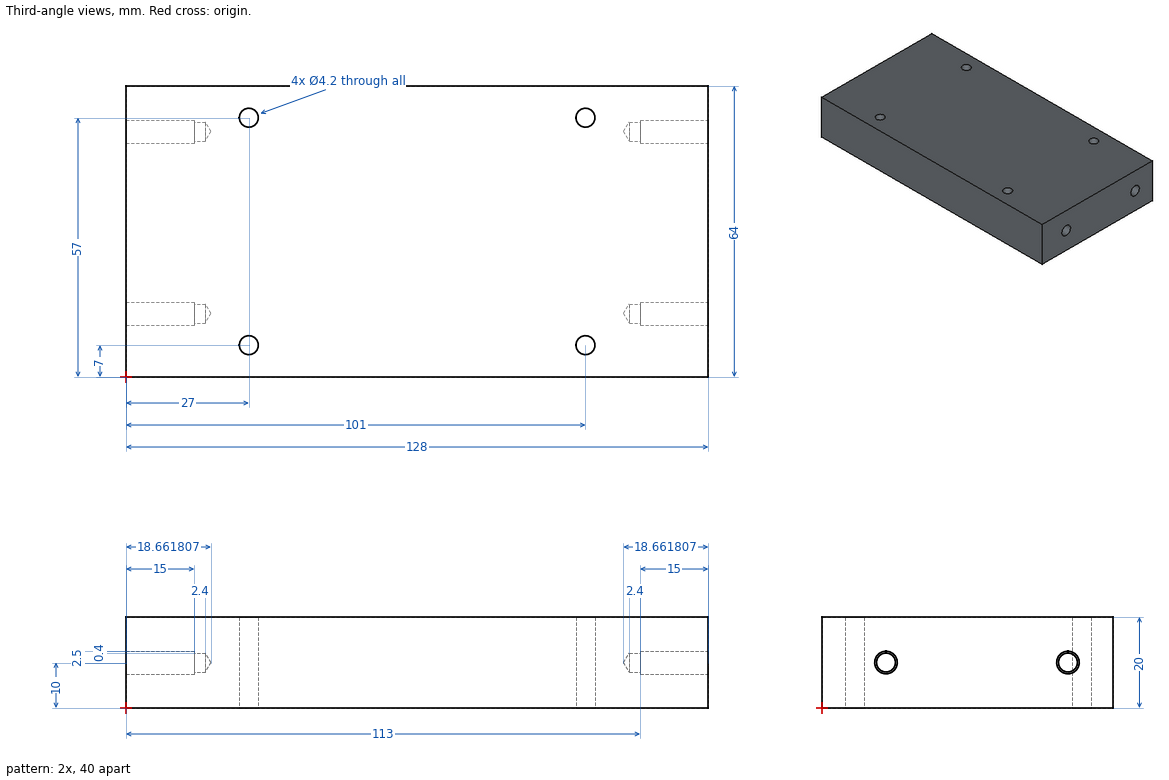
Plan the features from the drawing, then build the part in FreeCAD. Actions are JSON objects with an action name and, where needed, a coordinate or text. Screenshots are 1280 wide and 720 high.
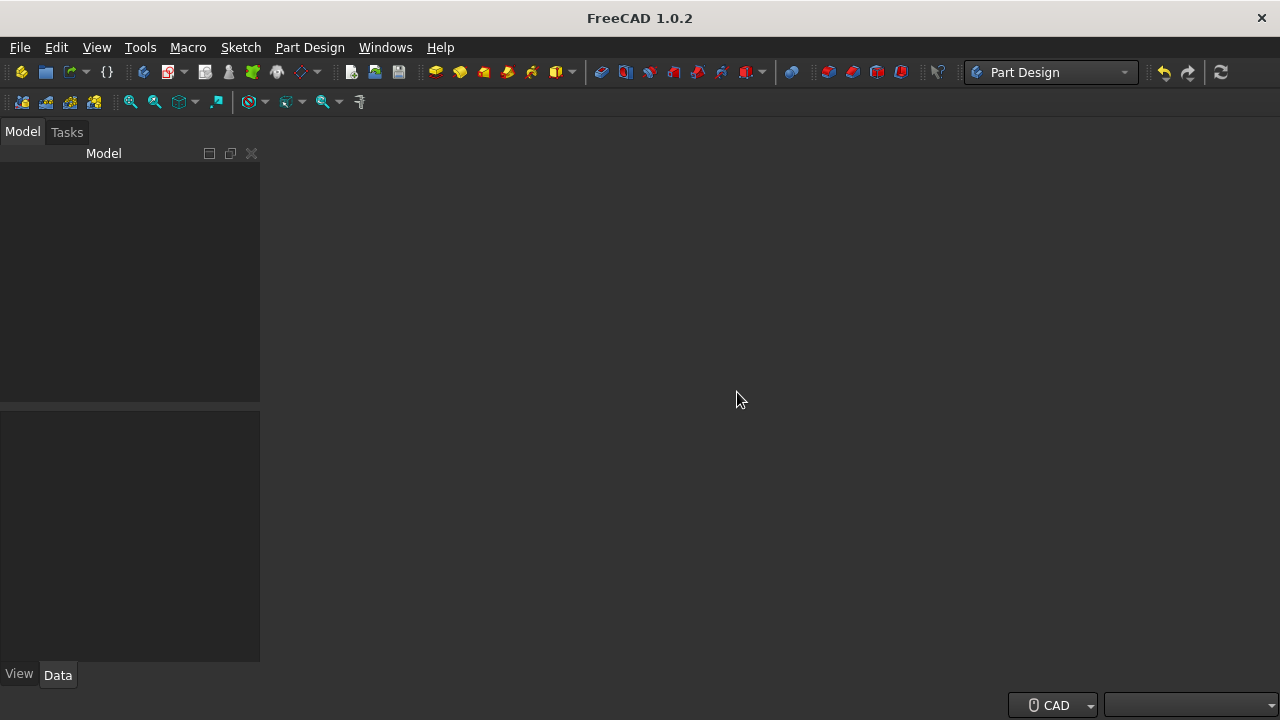
{"action": "left_click", "coordinate": [352, 72]}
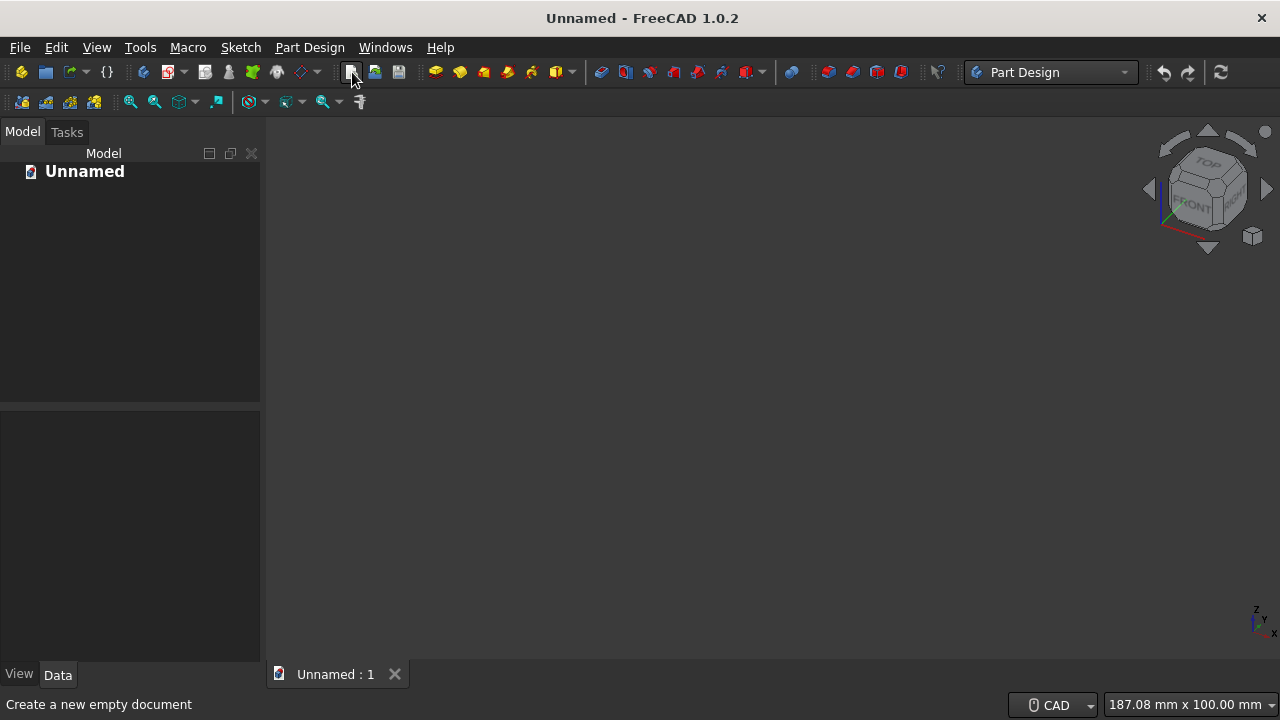
{"action": "left_click", "coordinate": [168, 72]}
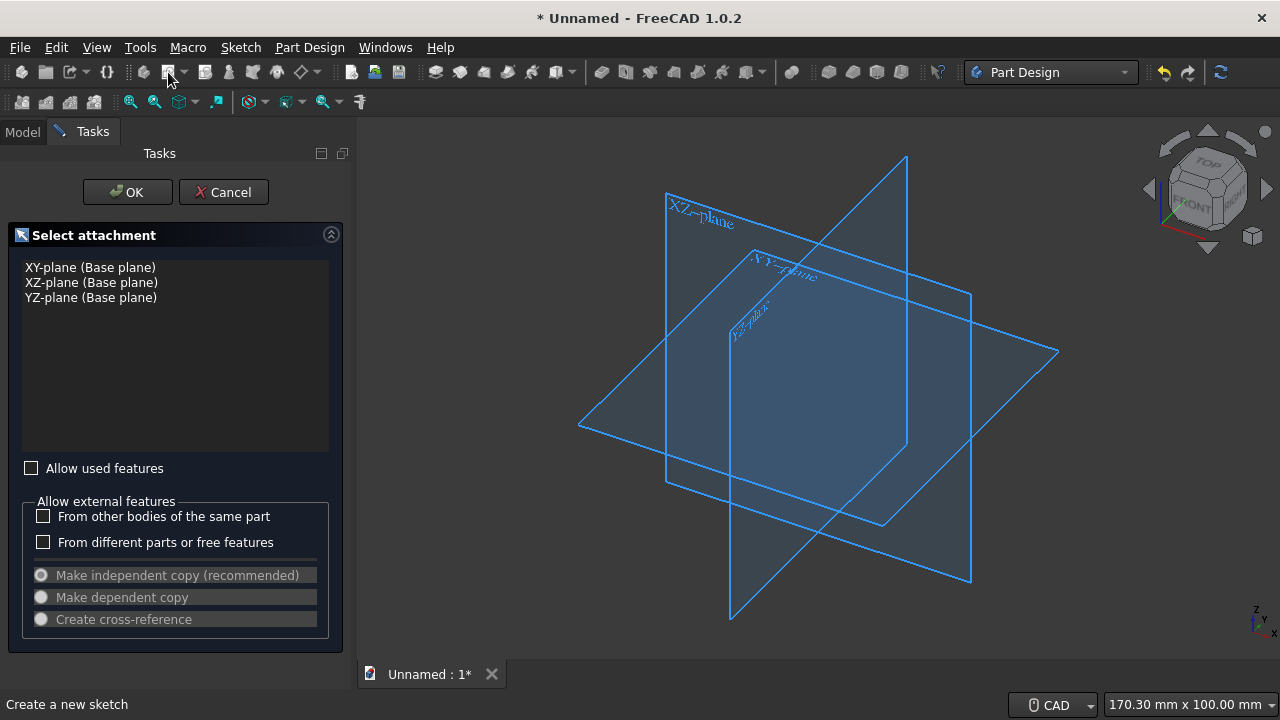
{"action": "left_click", "coordinate": [82, 268]}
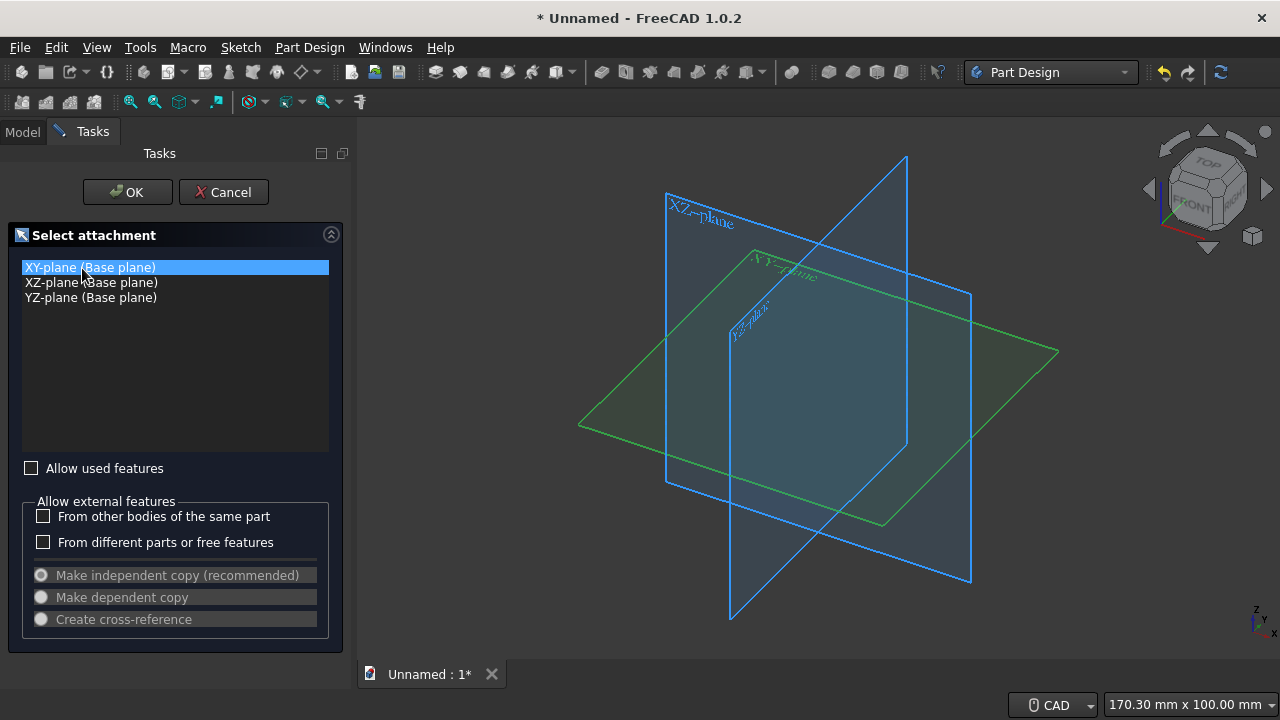
{"action": "left_click", "coordinate": [128, 192]}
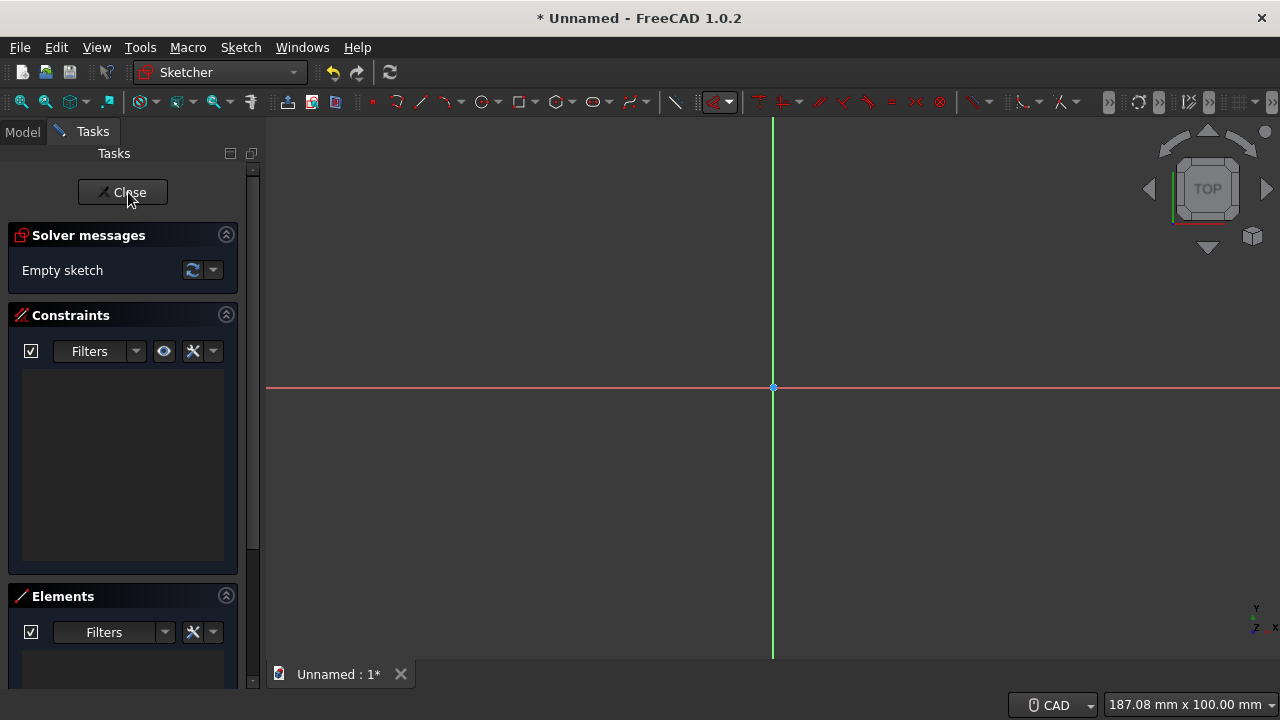
{"action": "scroll", "coordinate": [294, 631], "scroll_direction": "down", "scroll_amount": 2}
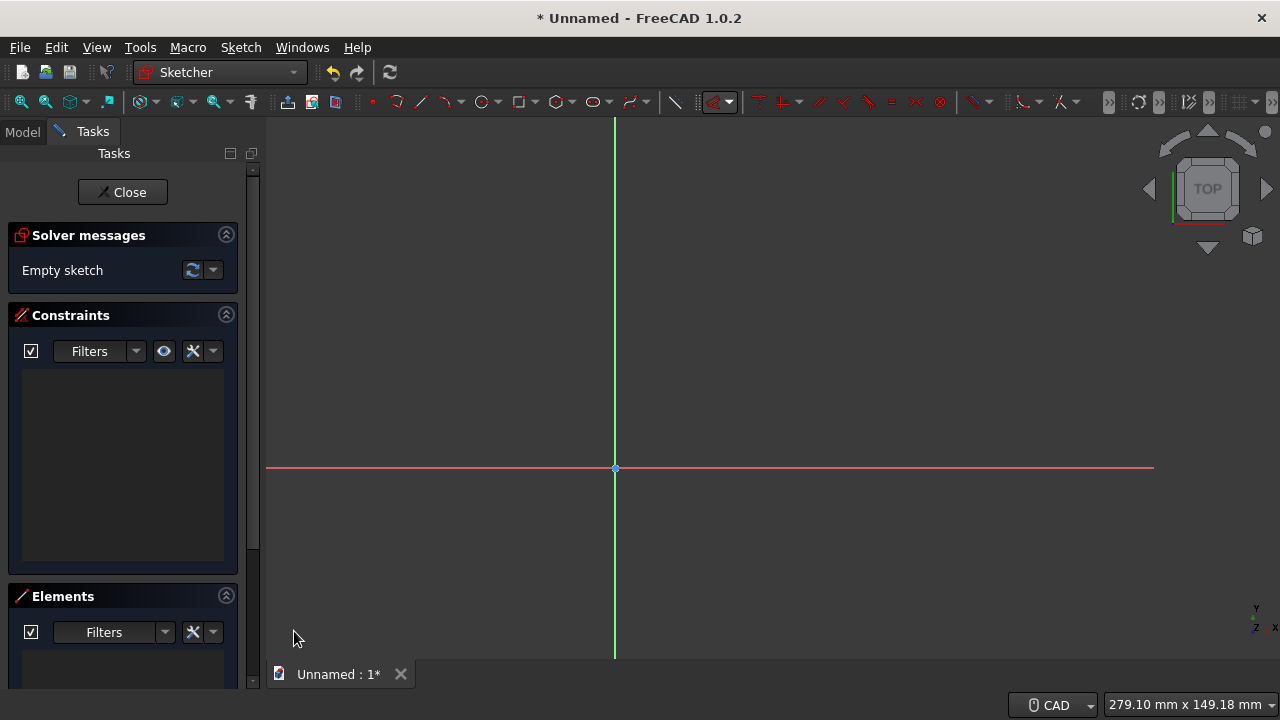
{"action": "left_click", "coordinate": [520, 102]}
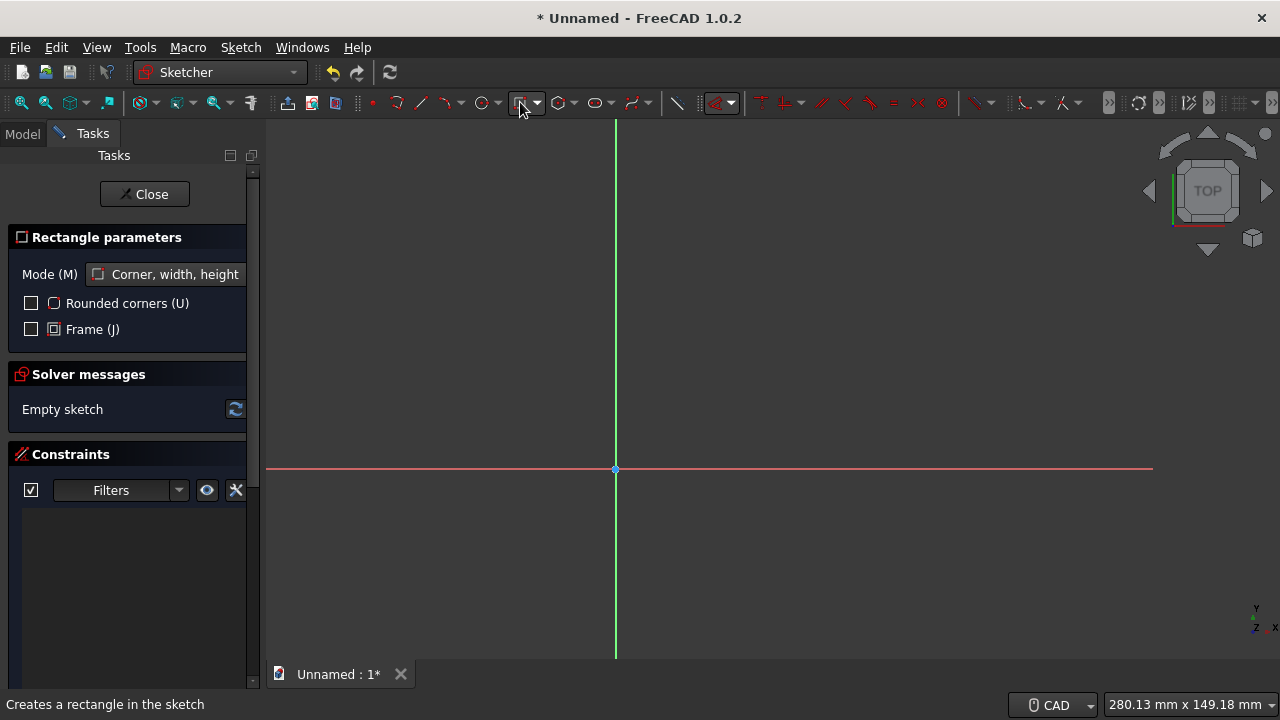
{"action": "left_click", "coordinate": [616, 469]}
{"action": "left_click", "coordinate": [1079, 237]}
{"action": "key", "text": "Escape"}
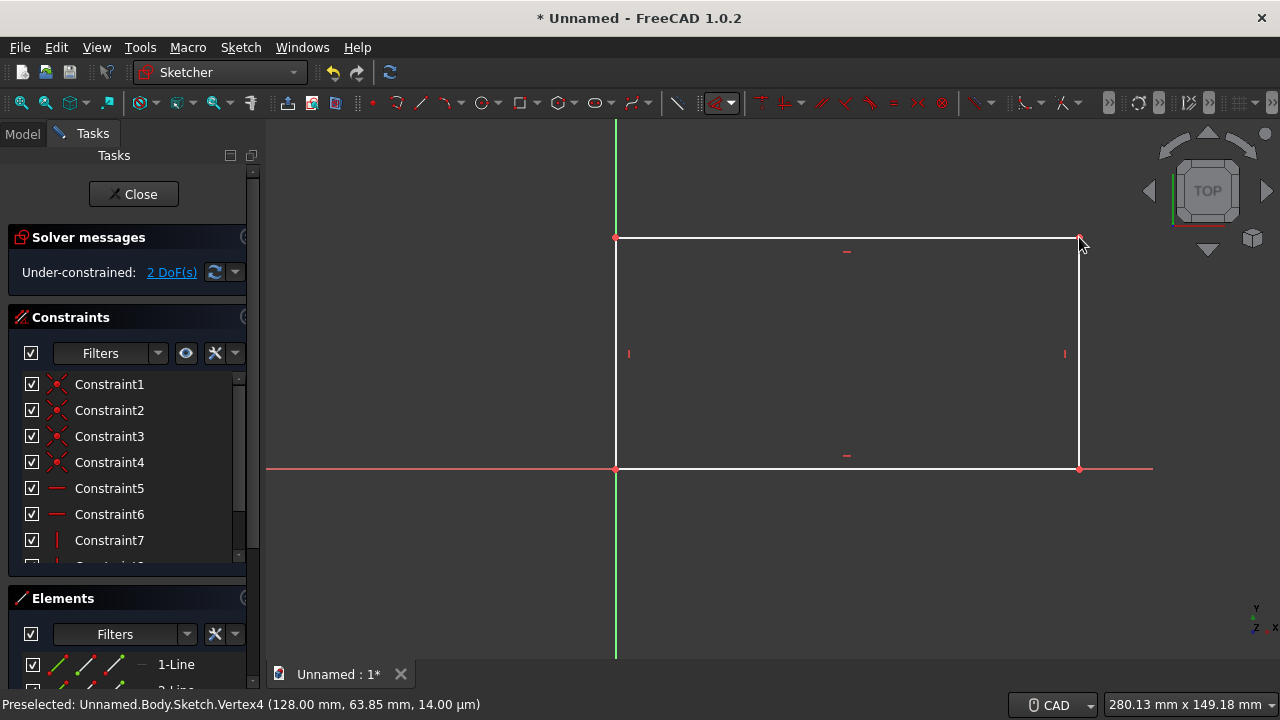
{"action": "left_click", "coordinate": [1079, 400]}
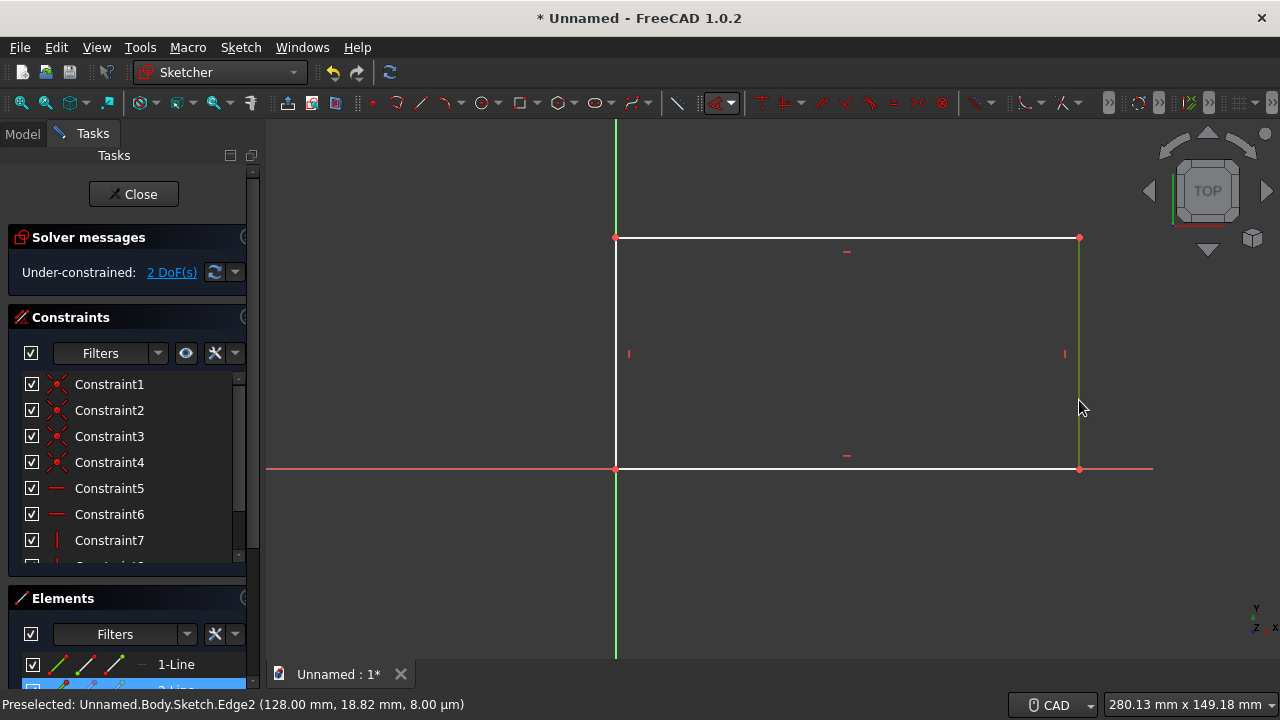
{"action": "key", "text": "i"}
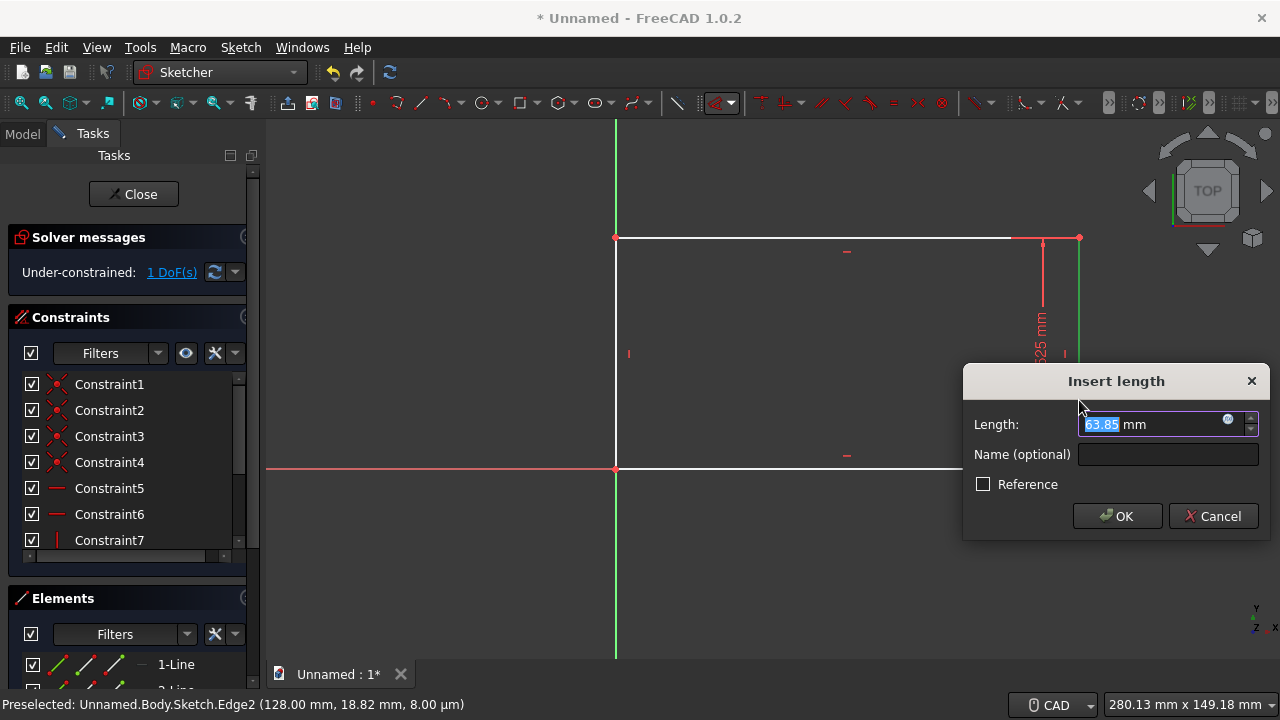
{"action": "type", "text": "64"}
{"action": "key", "text": "Return"}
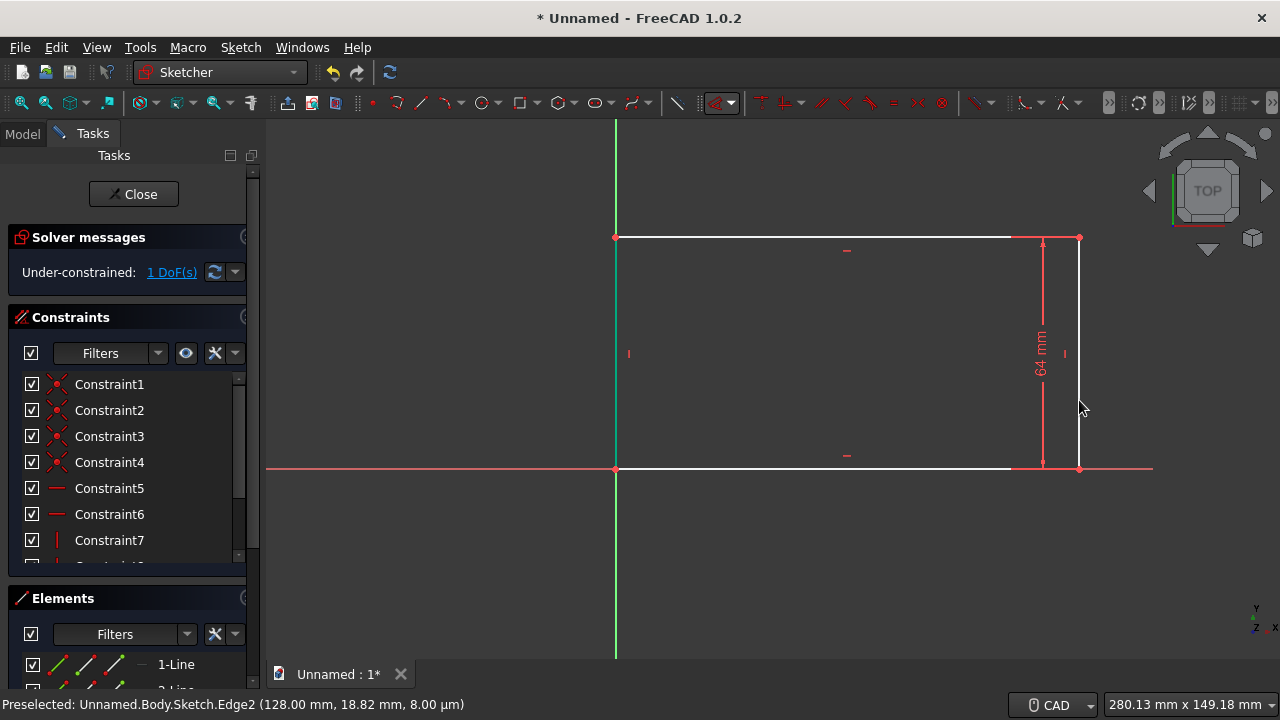
{"action": "left_click", "coordinate": [755, 469]}